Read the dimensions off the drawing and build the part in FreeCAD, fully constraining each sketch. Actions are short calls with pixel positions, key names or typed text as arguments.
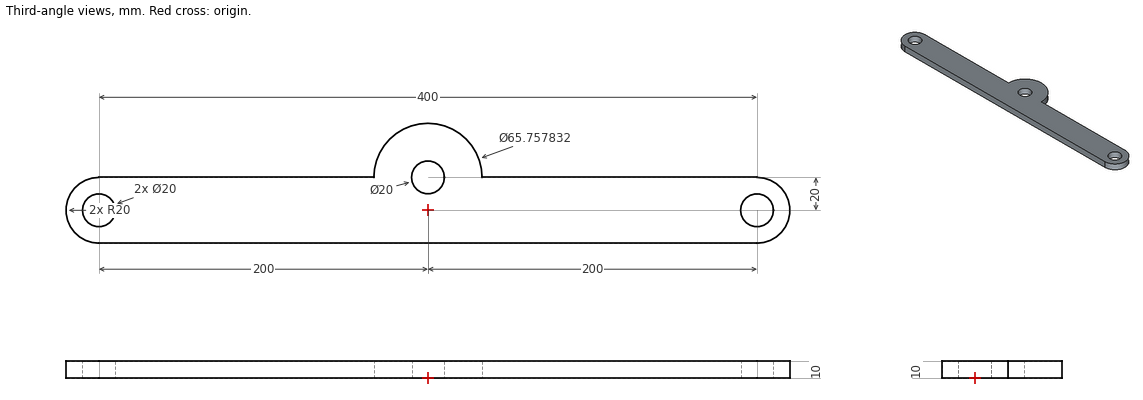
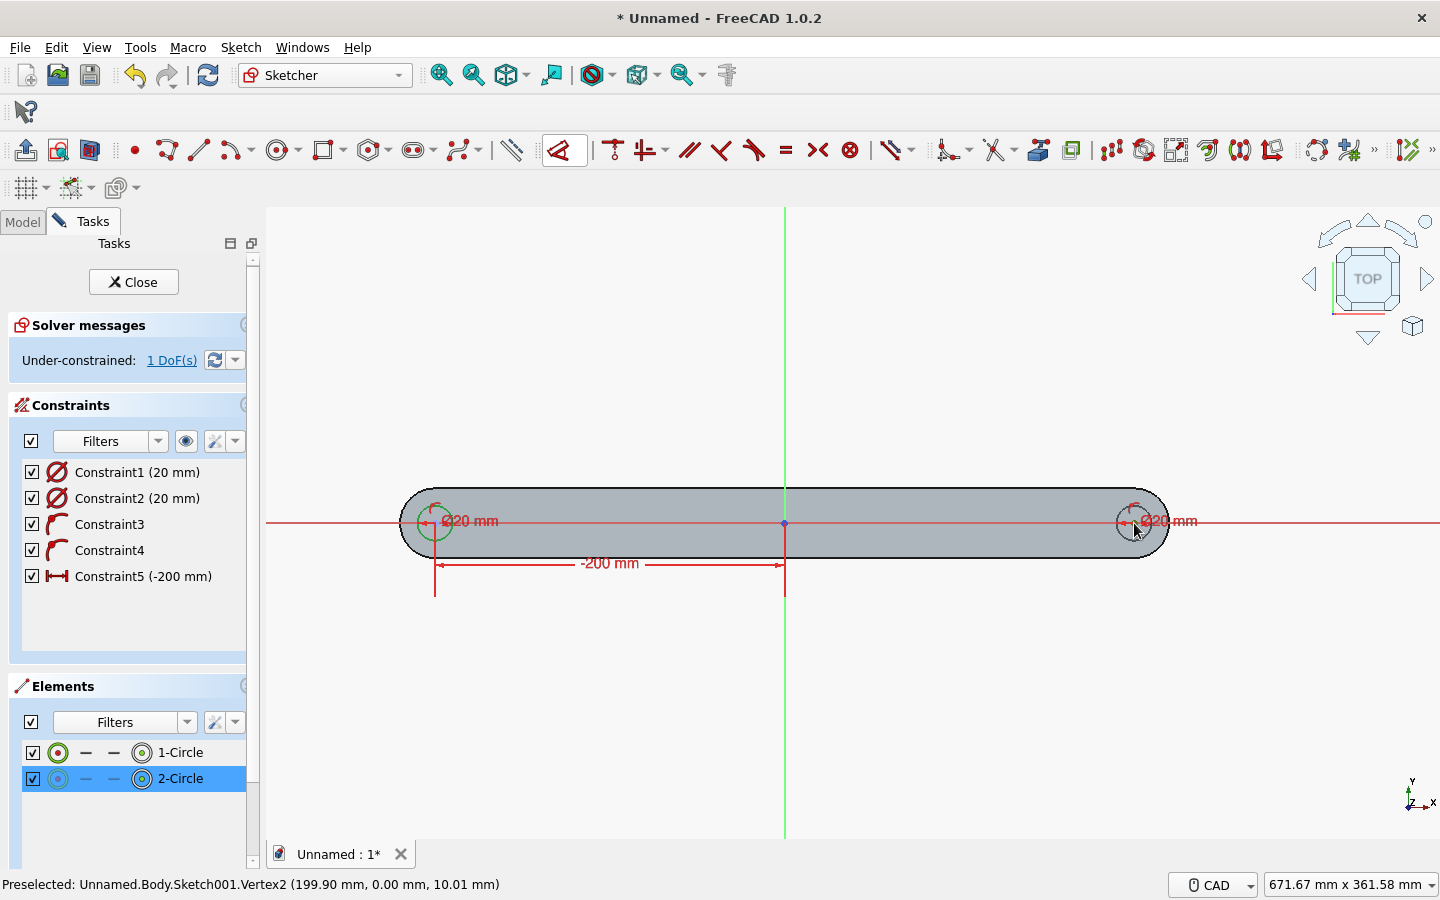
key(l)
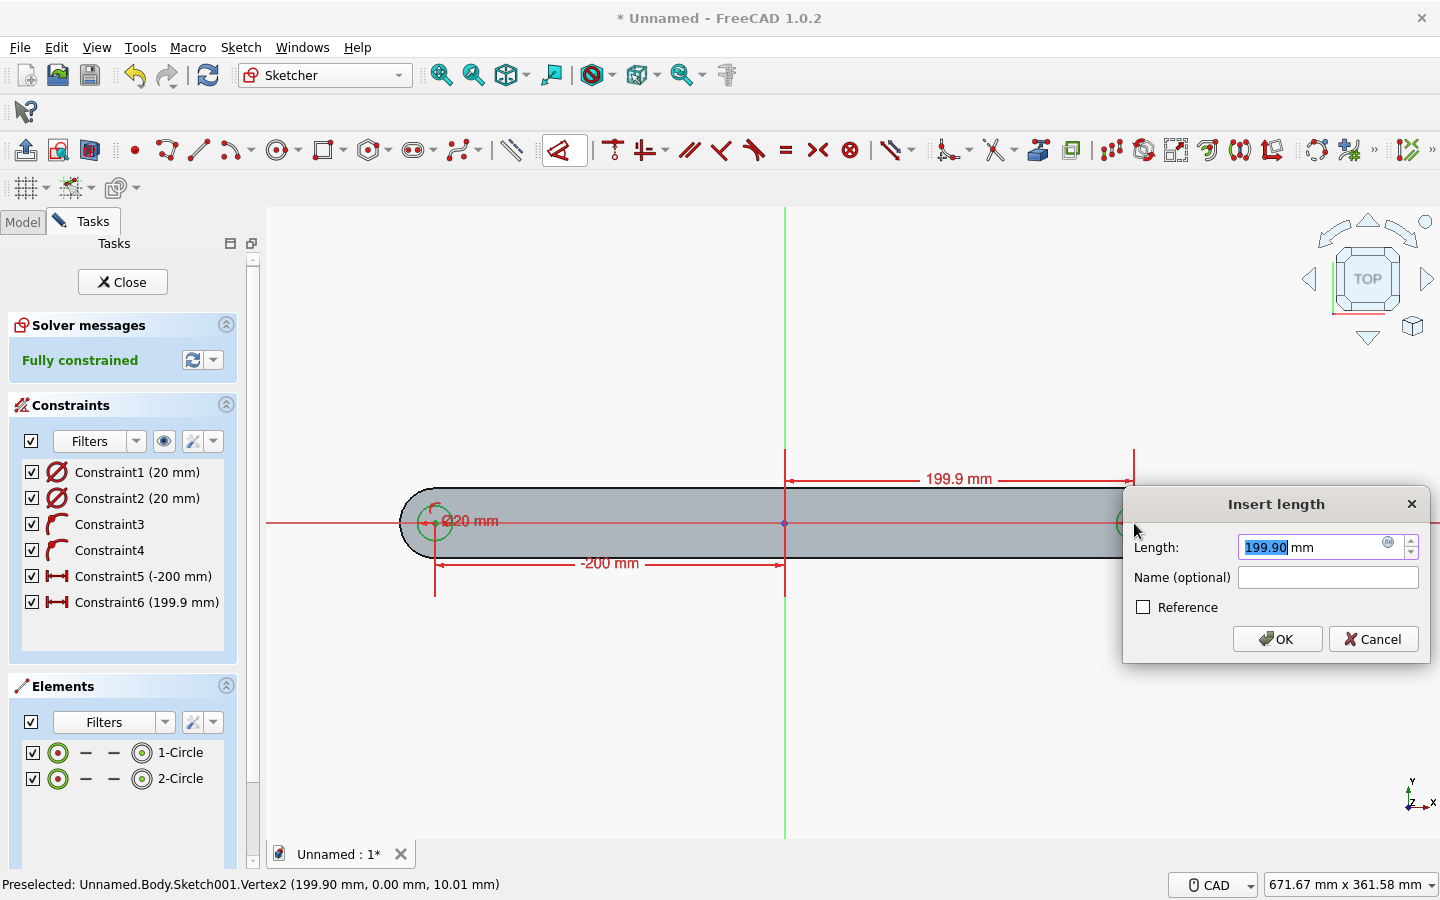
text(200)
key(Return)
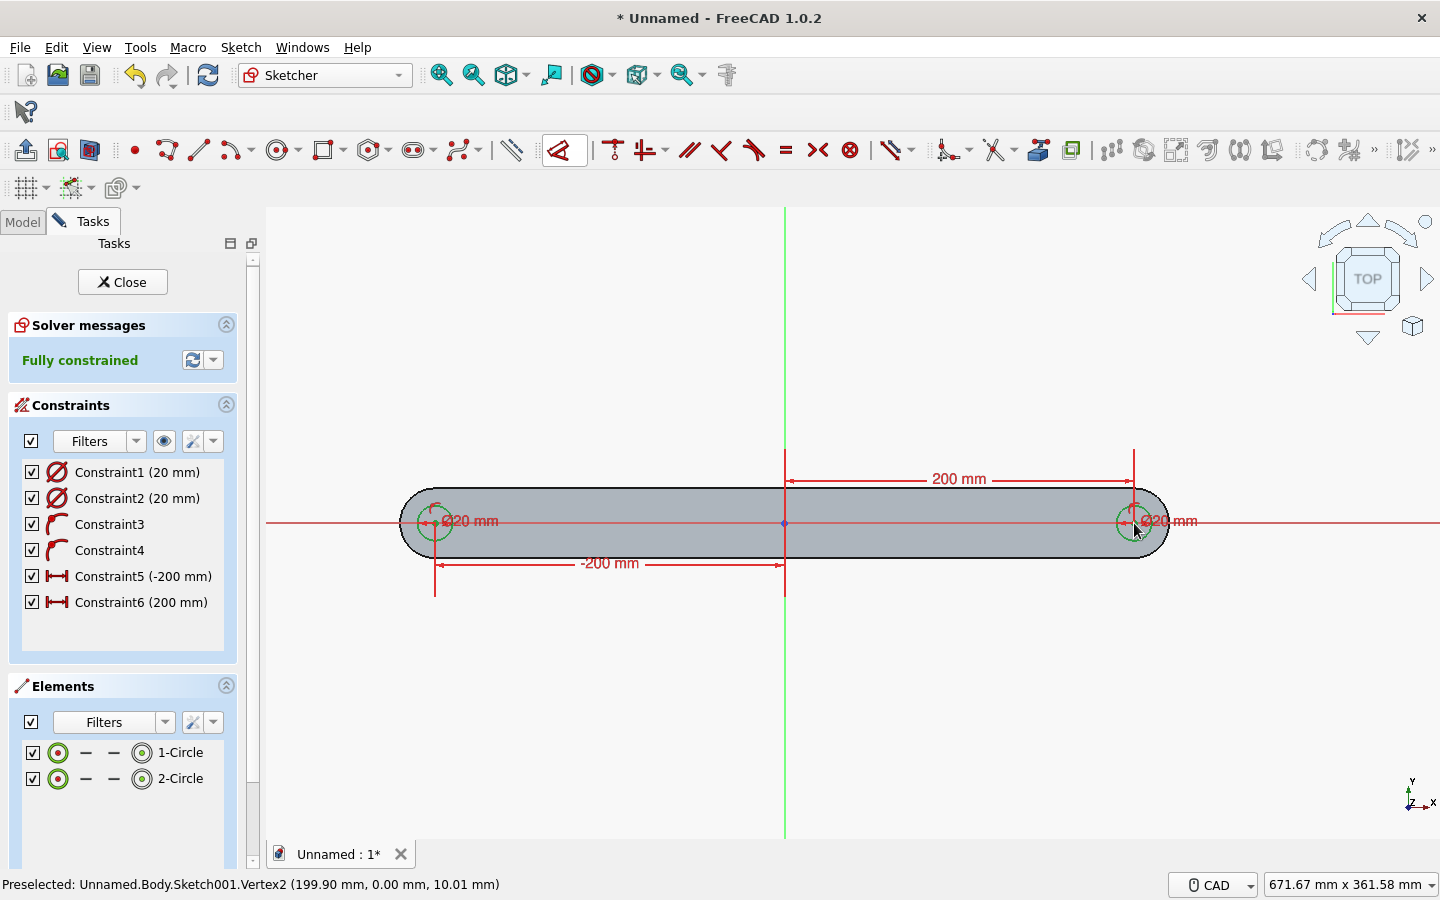
click(123, 282)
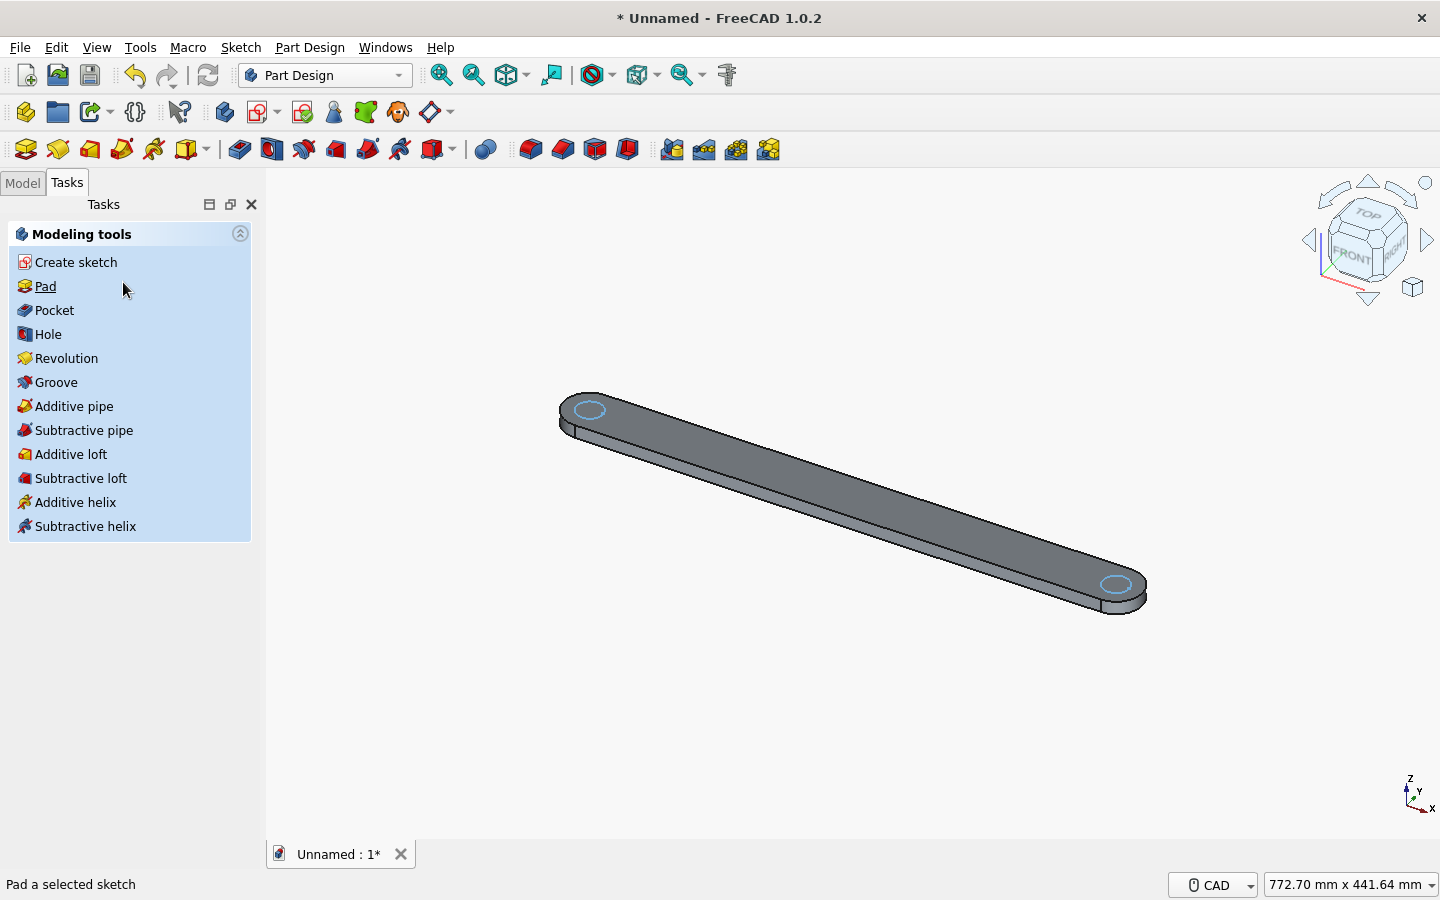
click(240, 150)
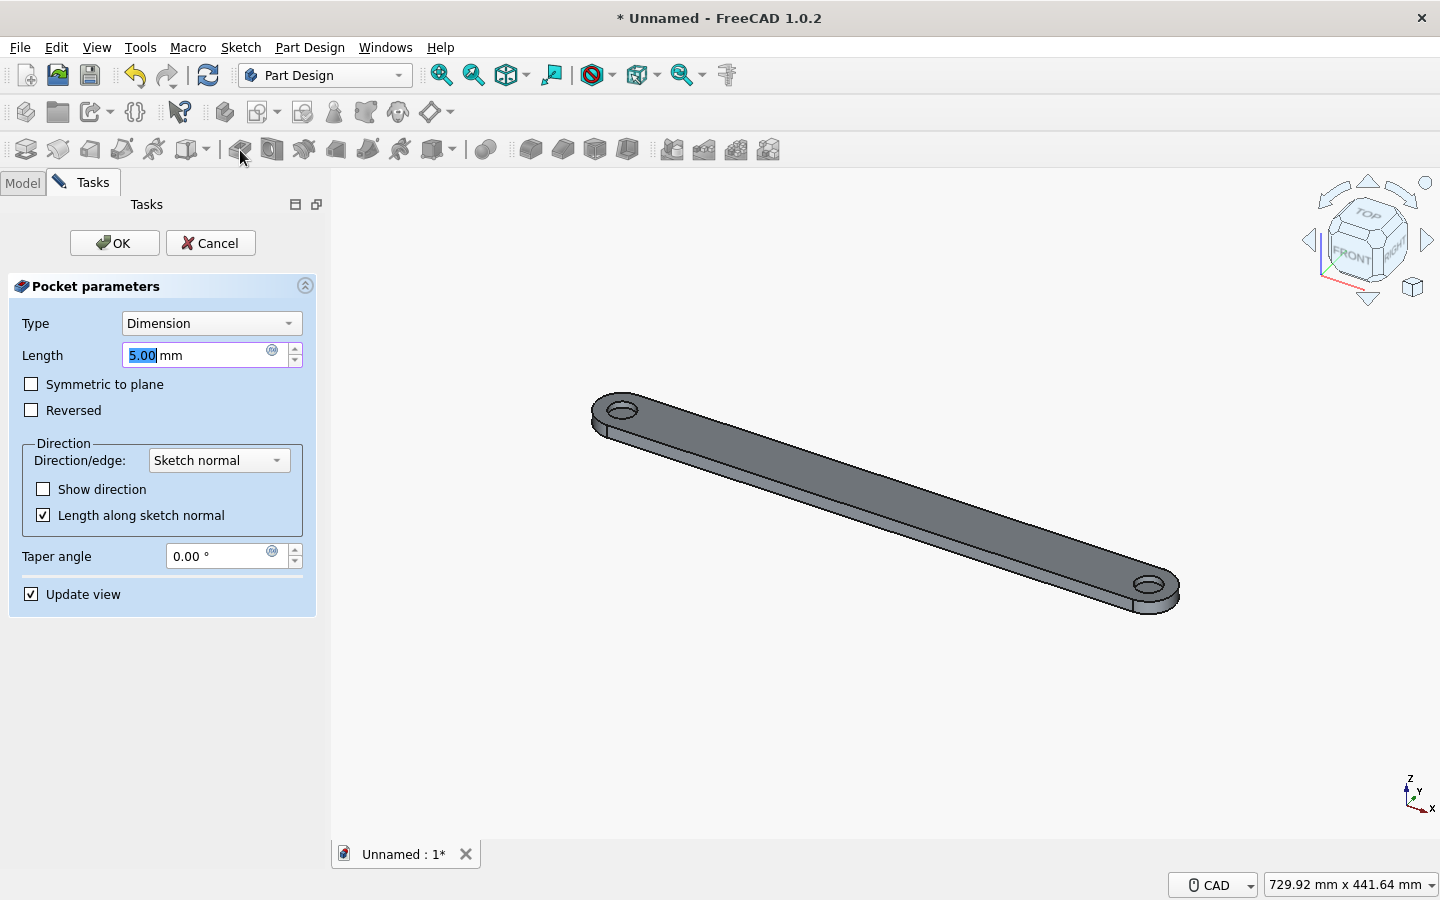
click(212, 324)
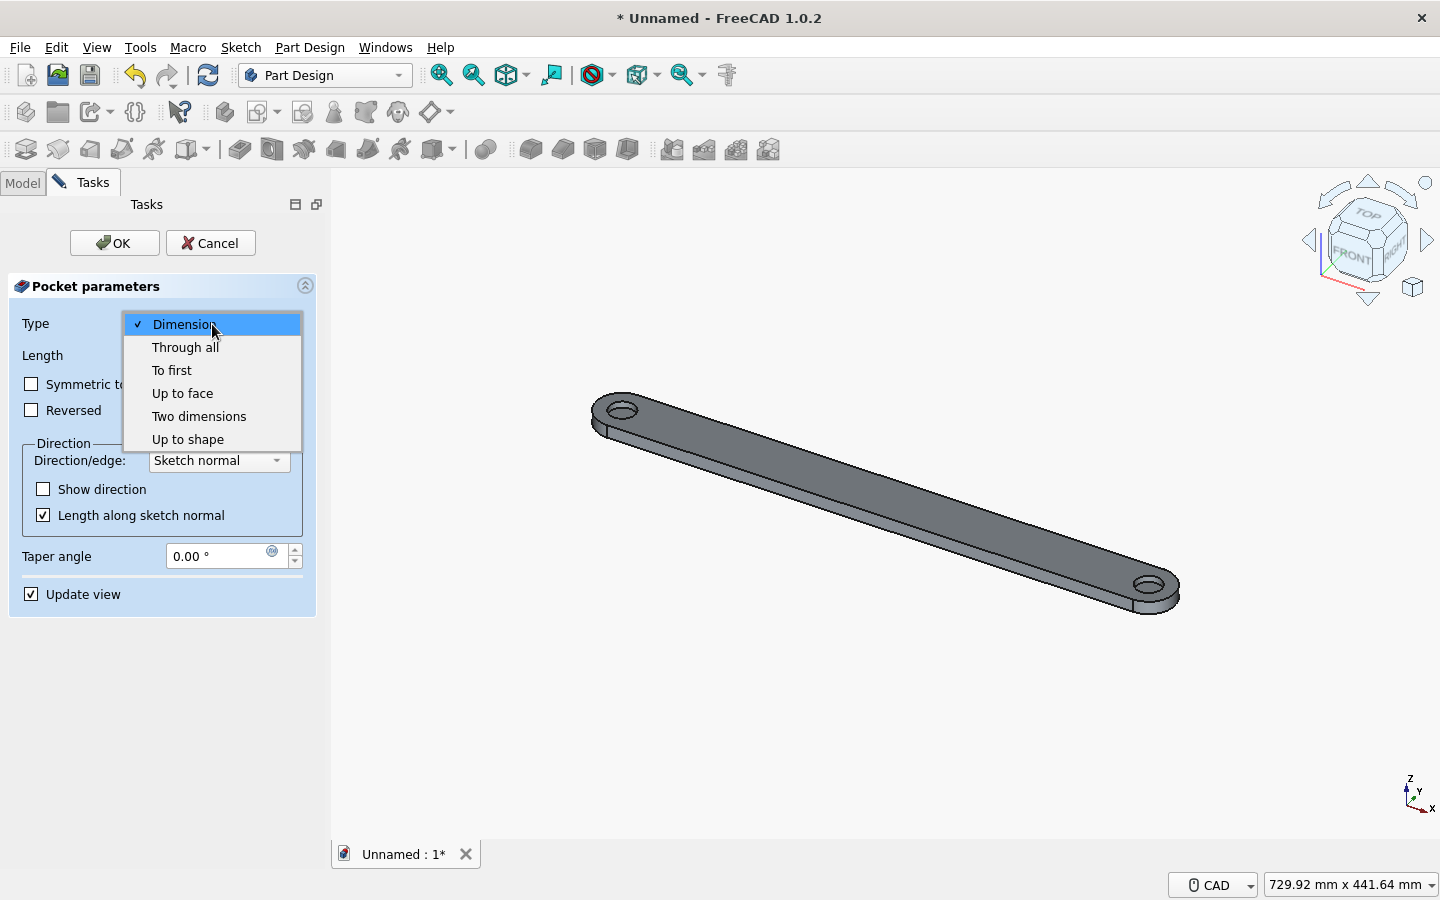
click(212, 348)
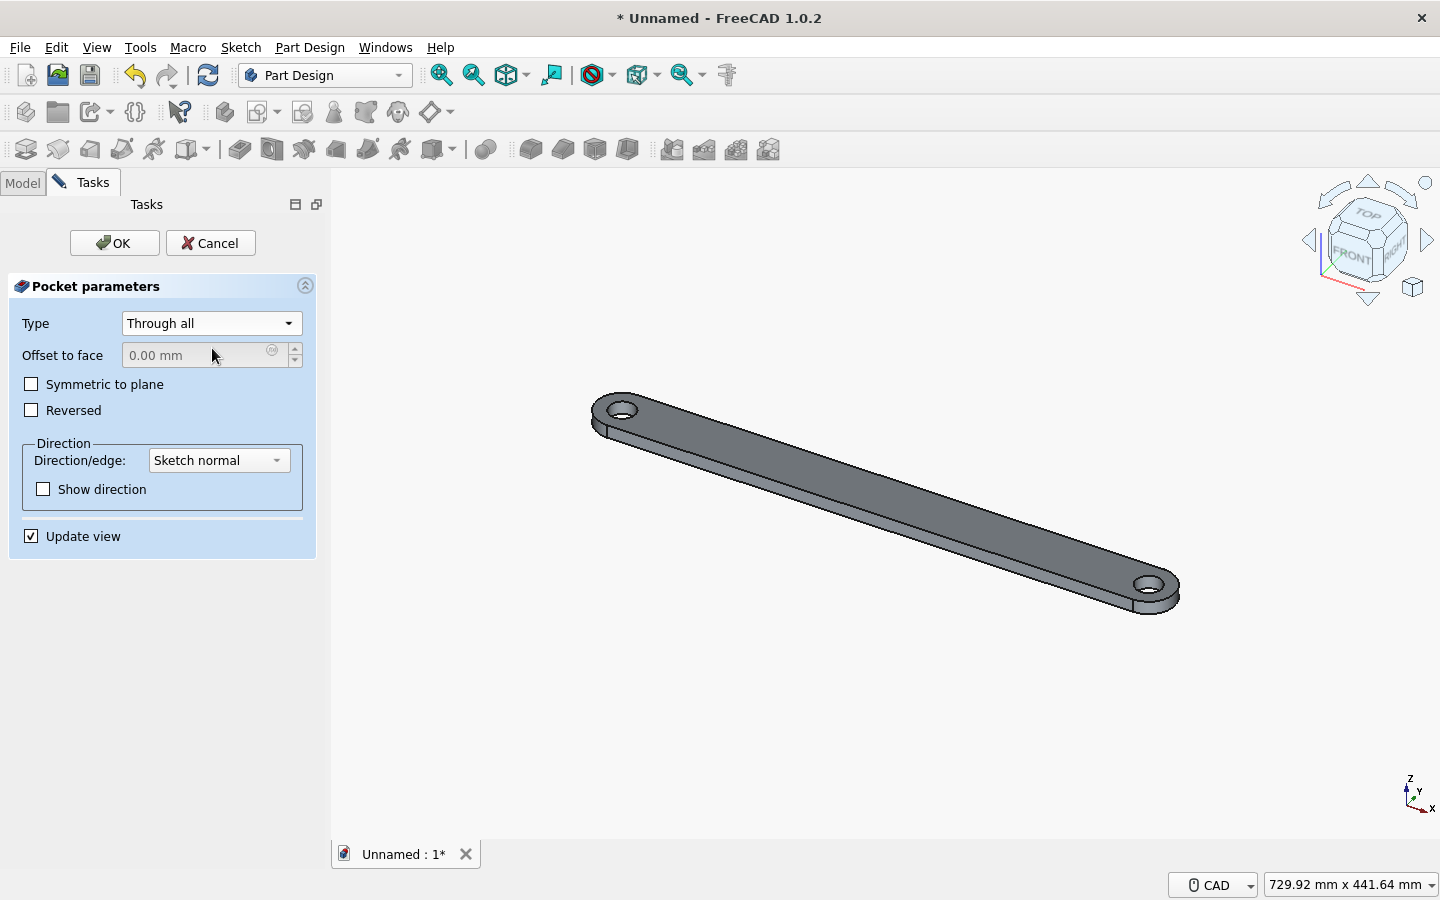
click(115, 243)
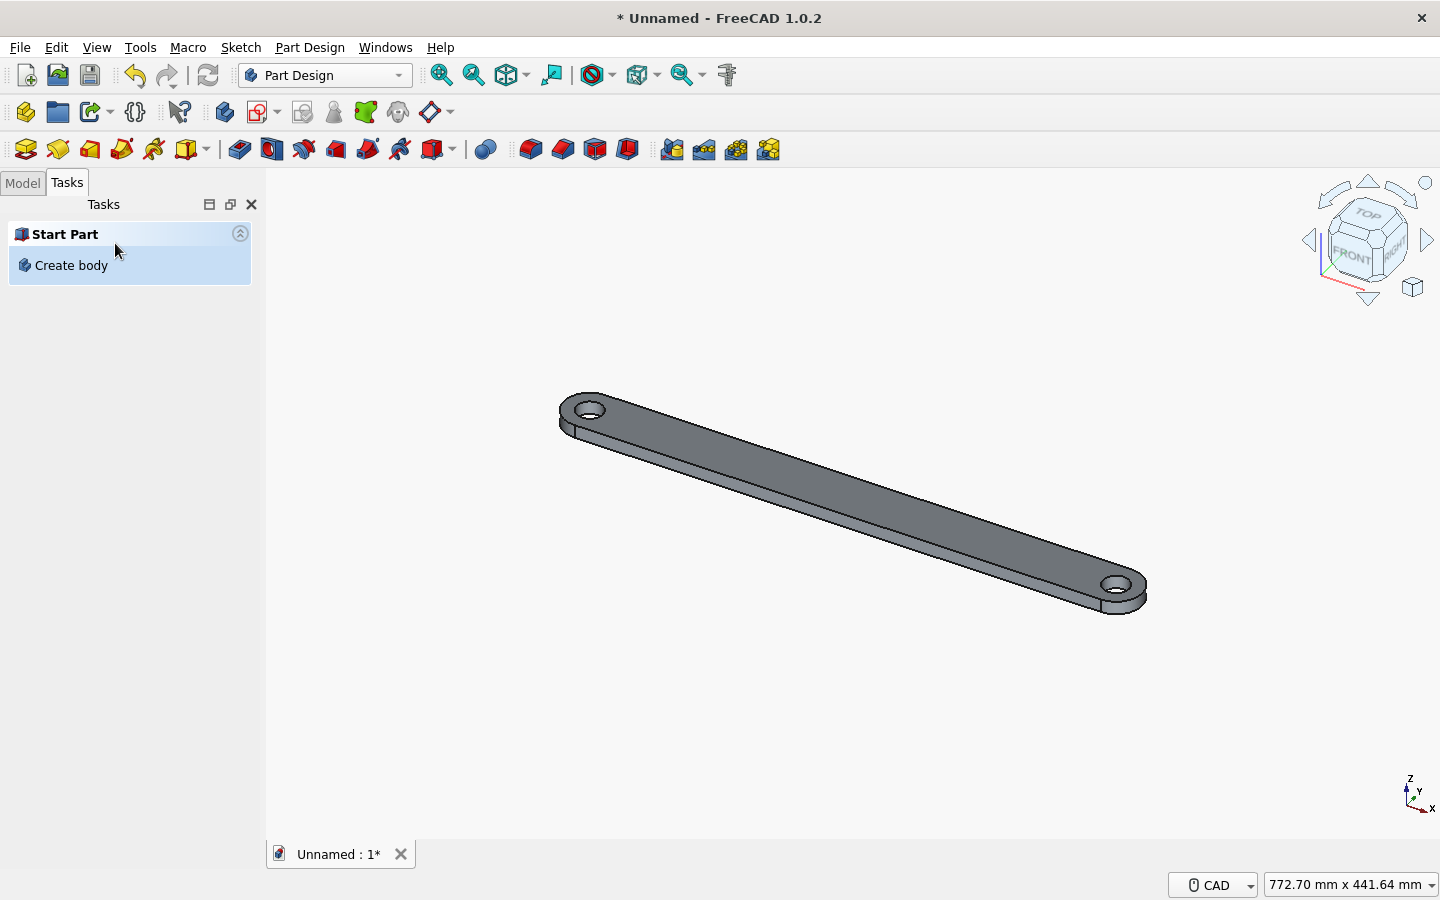
click(1018, 551)